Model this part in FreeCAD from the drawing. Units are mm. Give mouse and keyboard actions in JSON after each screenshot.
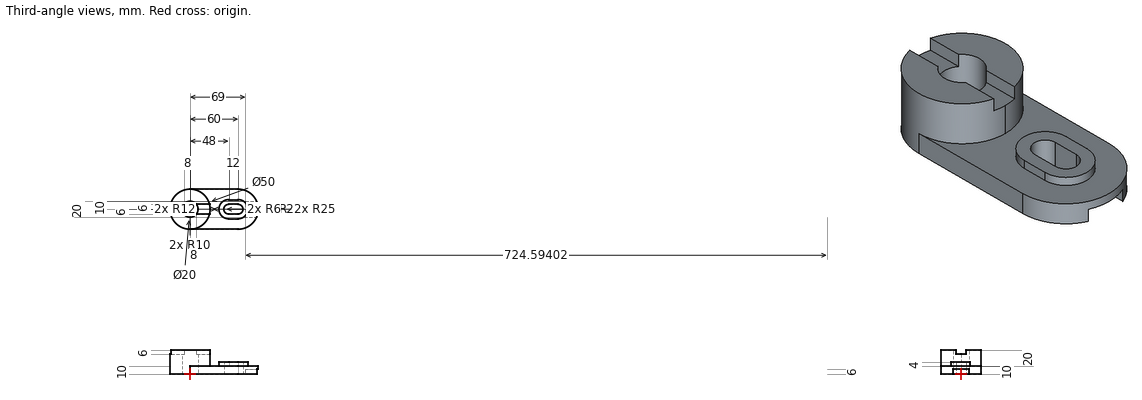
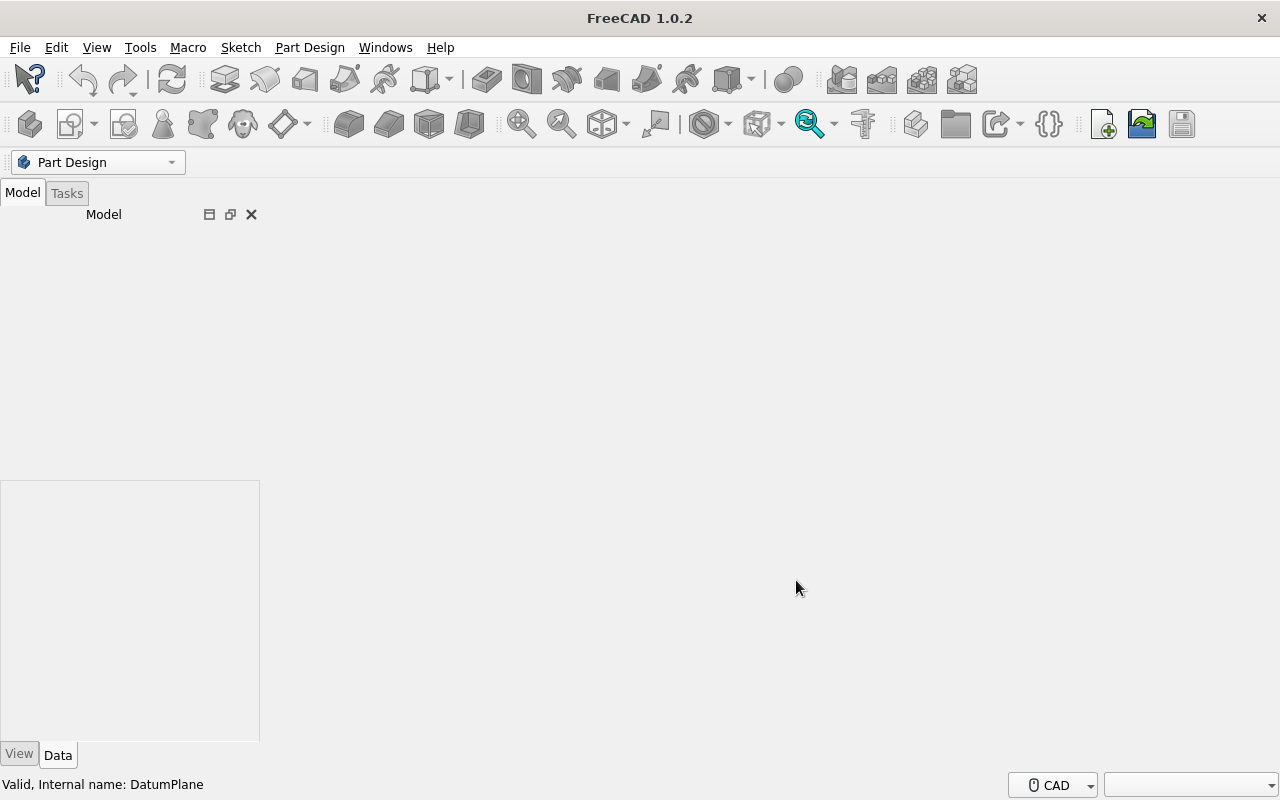
{"action": "left_click", "coordinate": [1102, 124]}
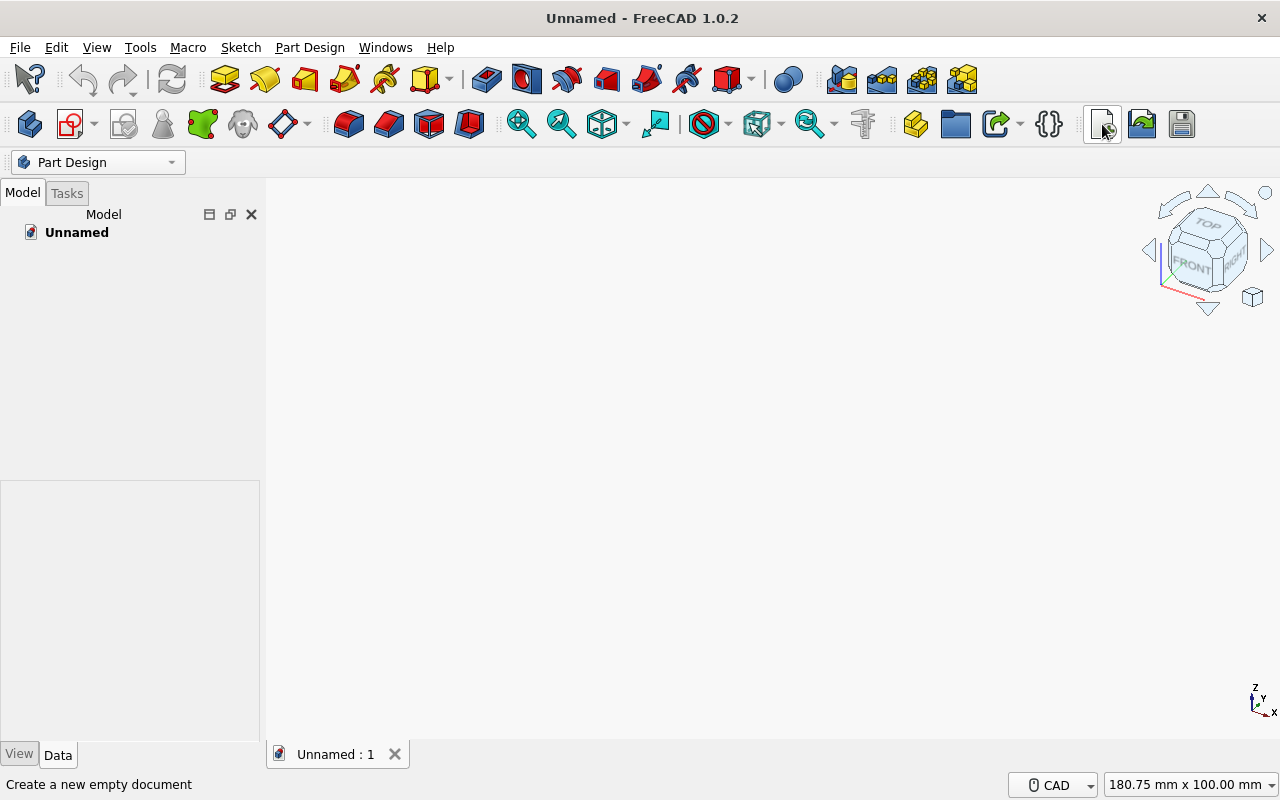
{"action": "left_click", "coordinate": [70, 124]}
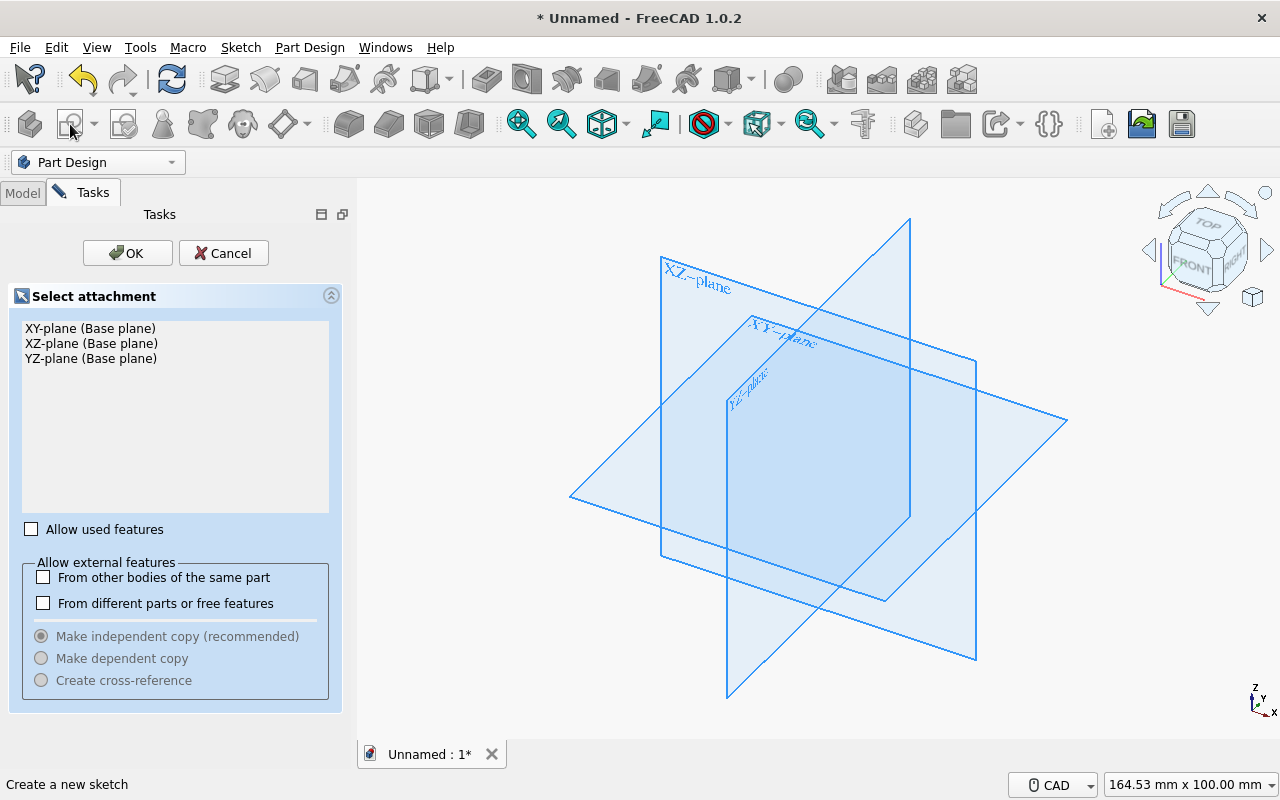
{"action": "left_click", "coordinate": [82, 328]}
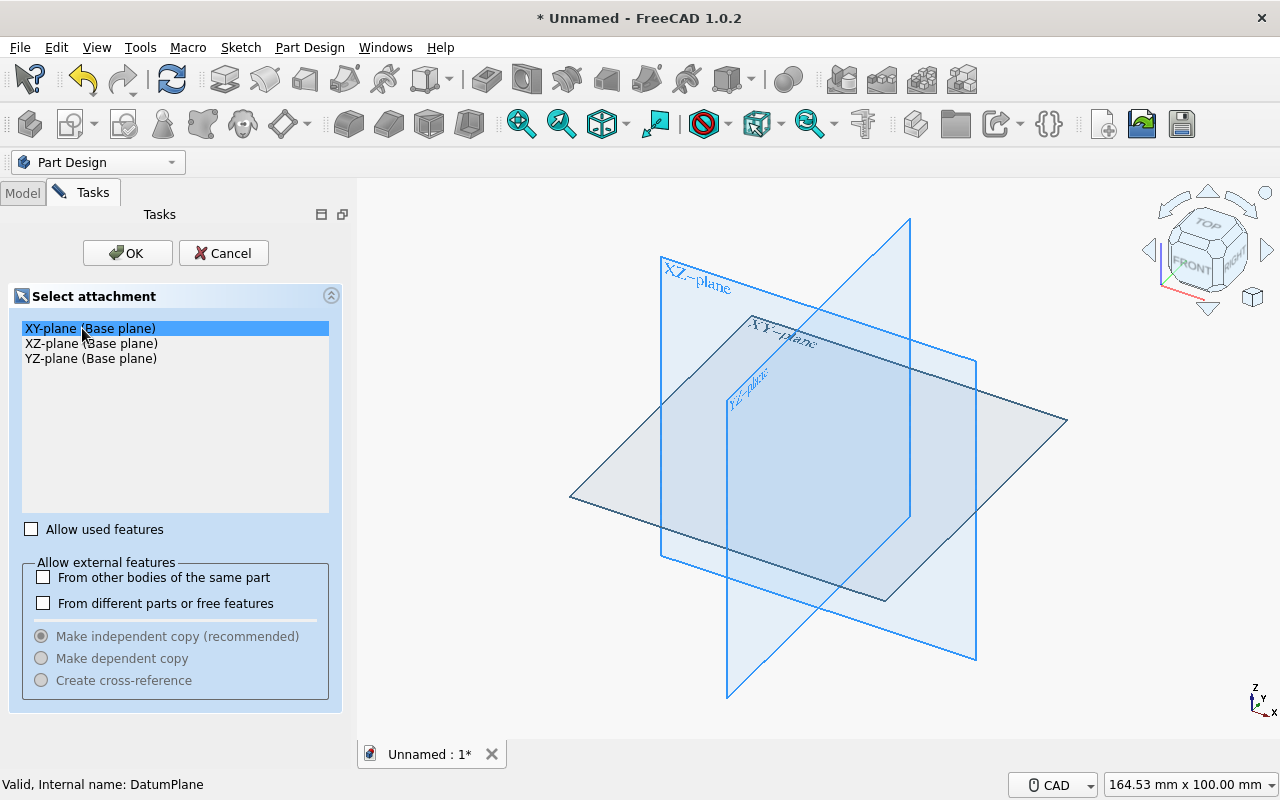
{"action": "left_click", "coordinate": [128, 253]}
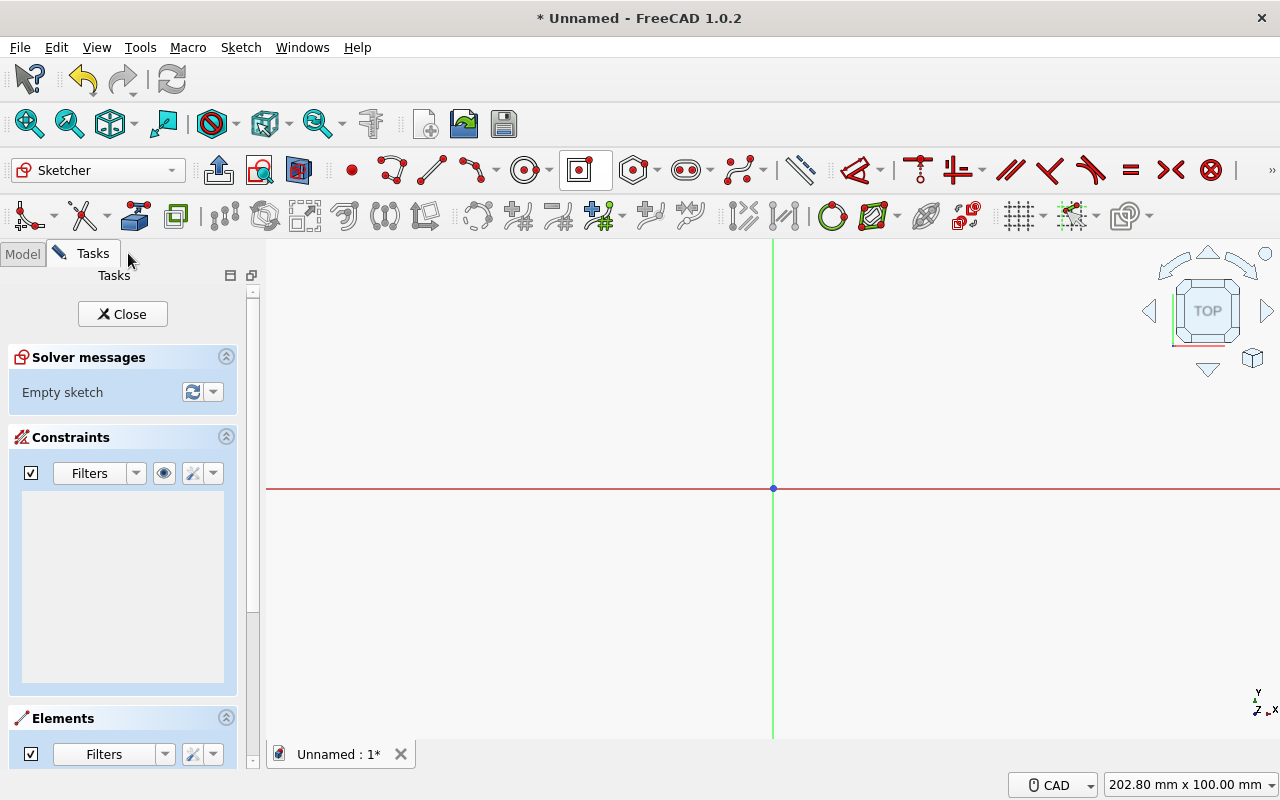
{"action": "scroll", "coordinate": [294, 489], "scroll_direction": "down", "scroll_amount": 1}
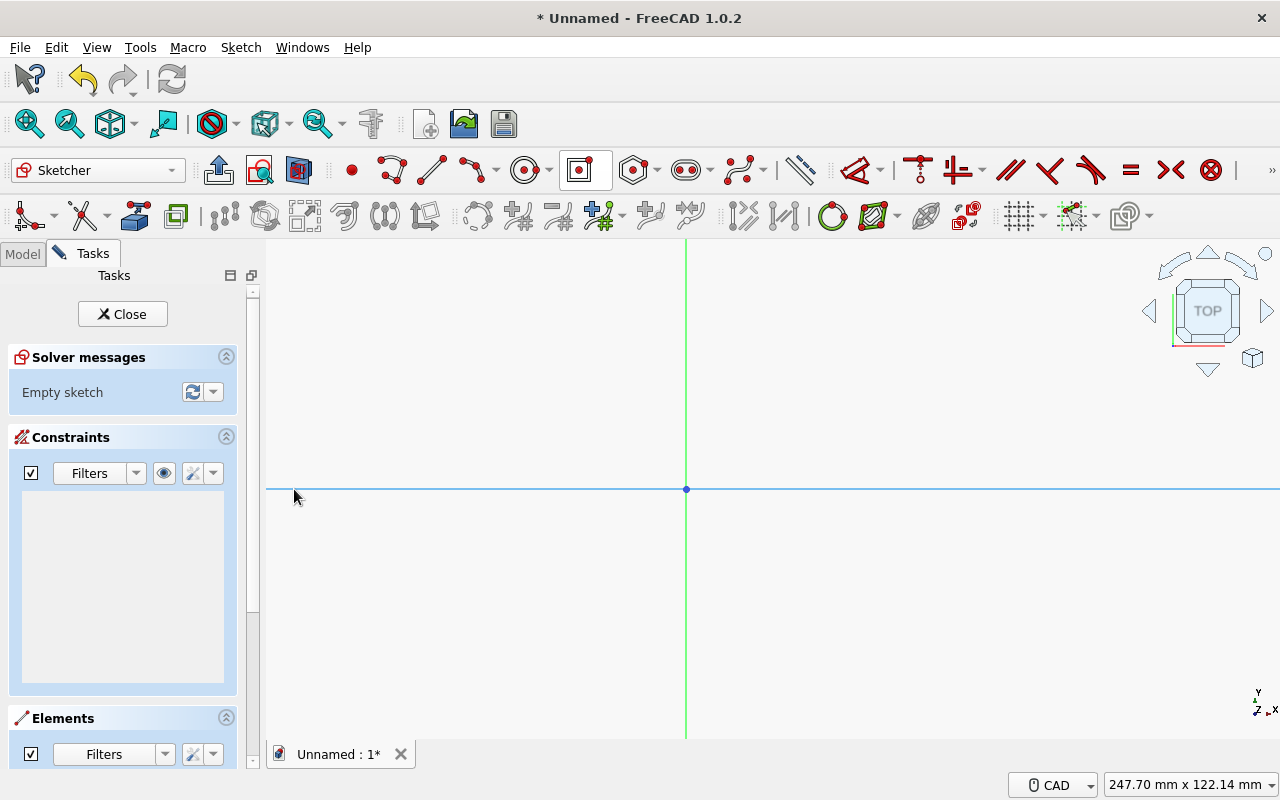
{"action": "scroll", "coordinate": [1115, 489], "scroll_direction": "up", "scroll_amount": 2}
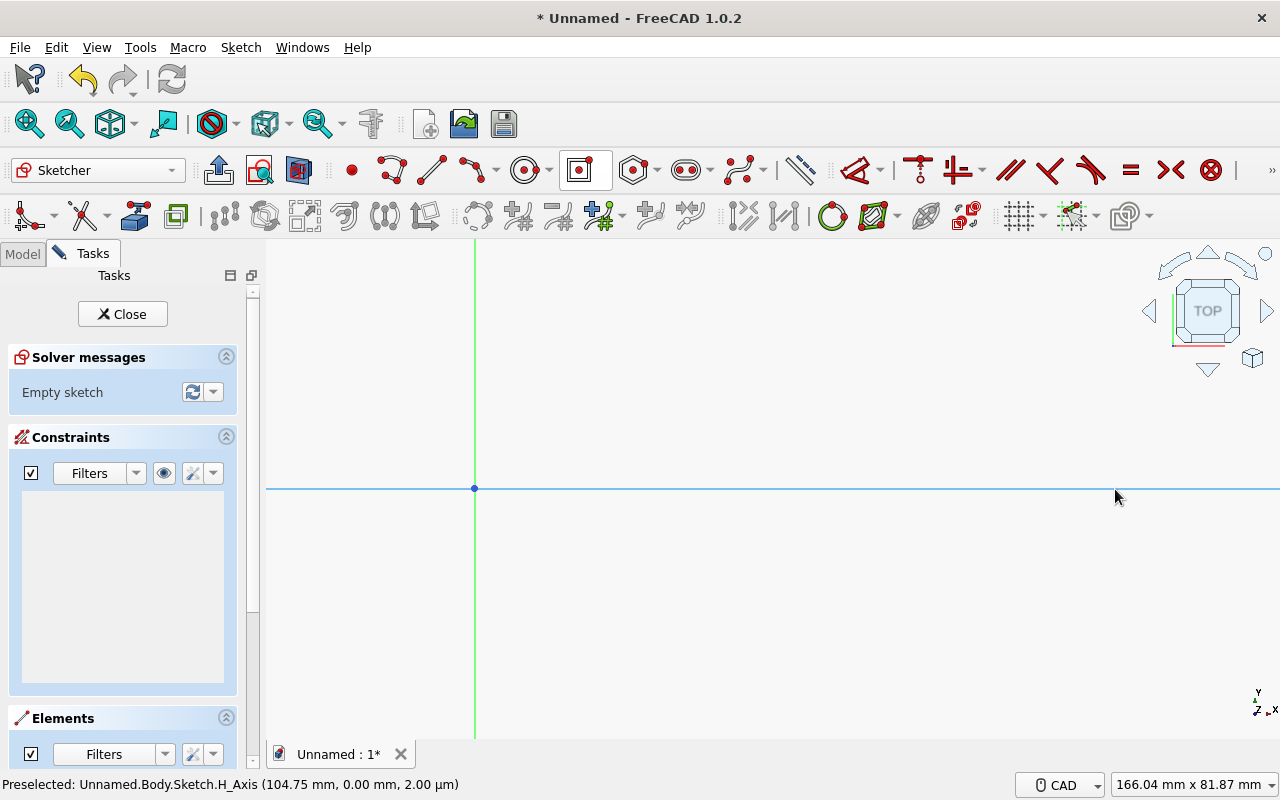
{"action": "left_click", "coordinate": [392, 170]}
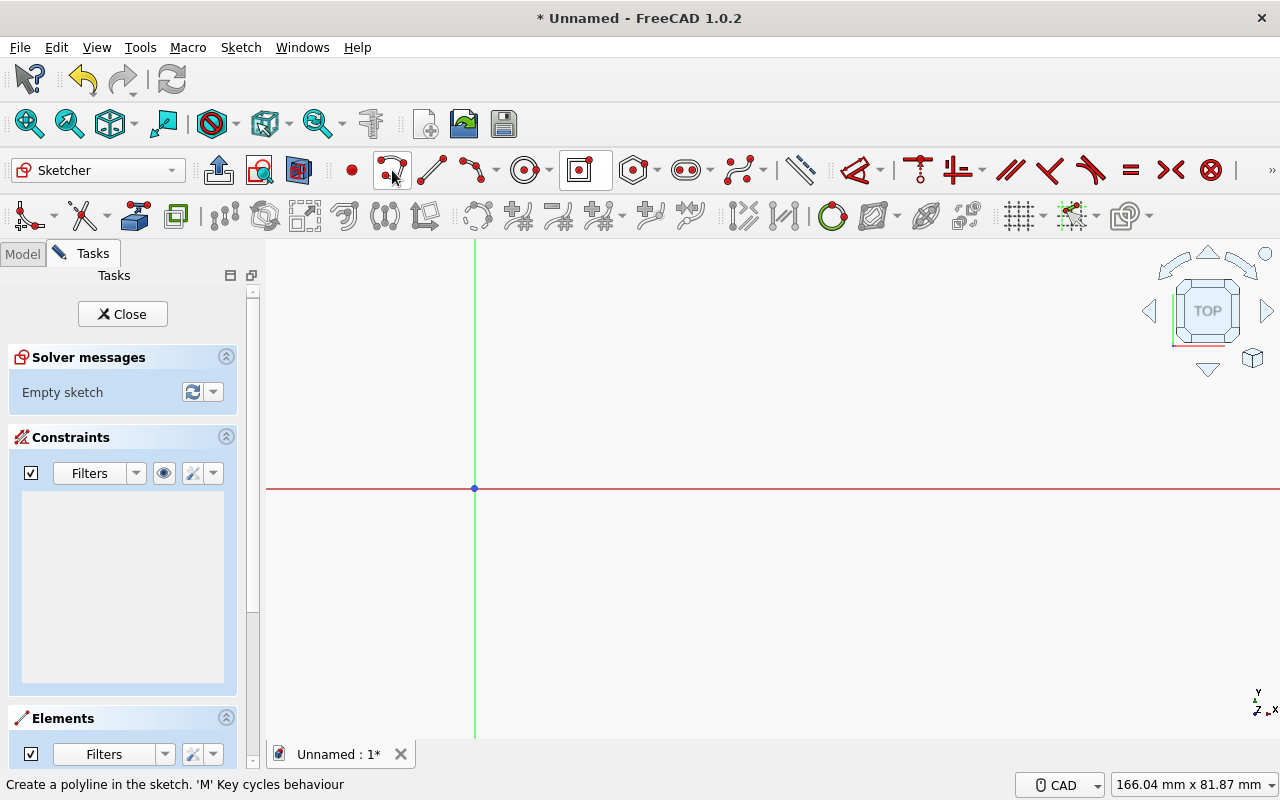
{"action": "left_click", "coordinate": [841, 336]}
{"action": "left_click", "coordinate": [475, 336]}
{"action": "left_click", "coordinate": [484, 642]}
{"action": "left_click", "coordinate": [841, 642]}
{"action": "right_click", "coordinate": [841, 642]}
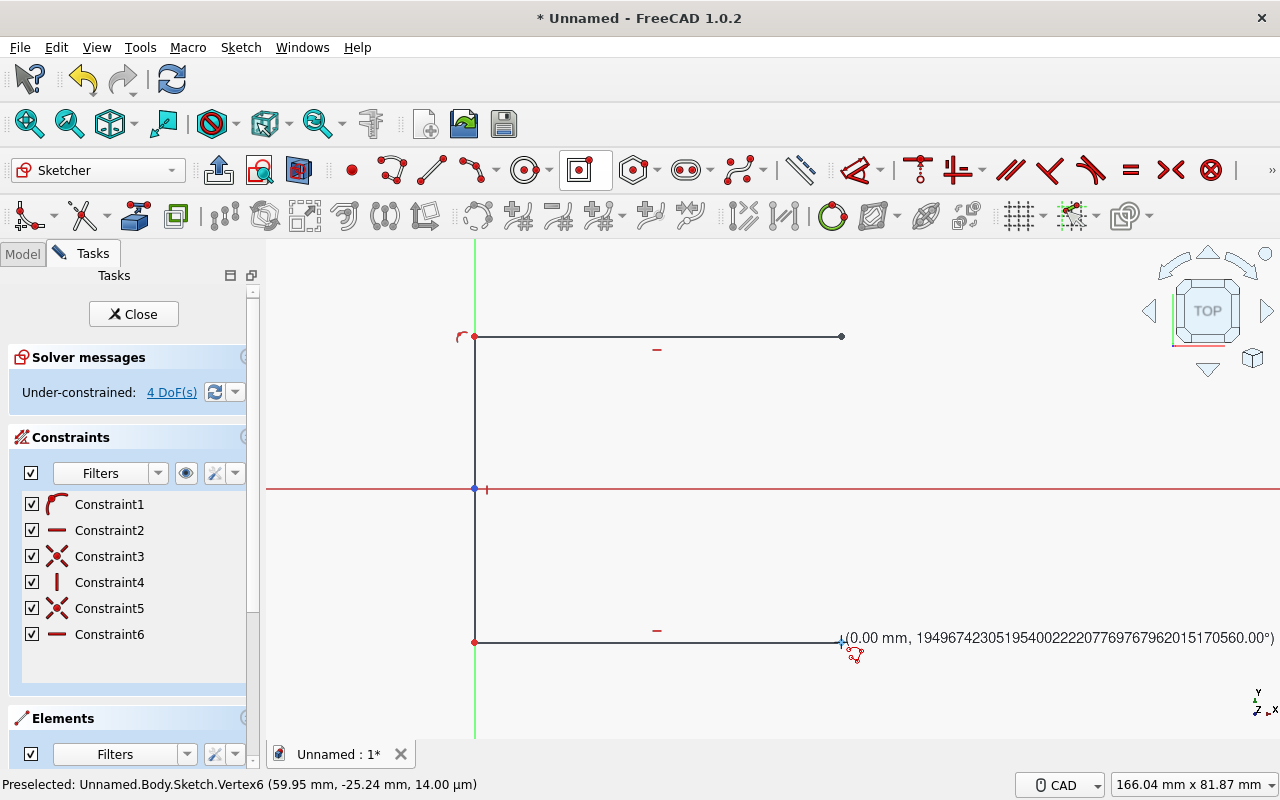
{"action": "left_click", "coordinate": [472, 170]}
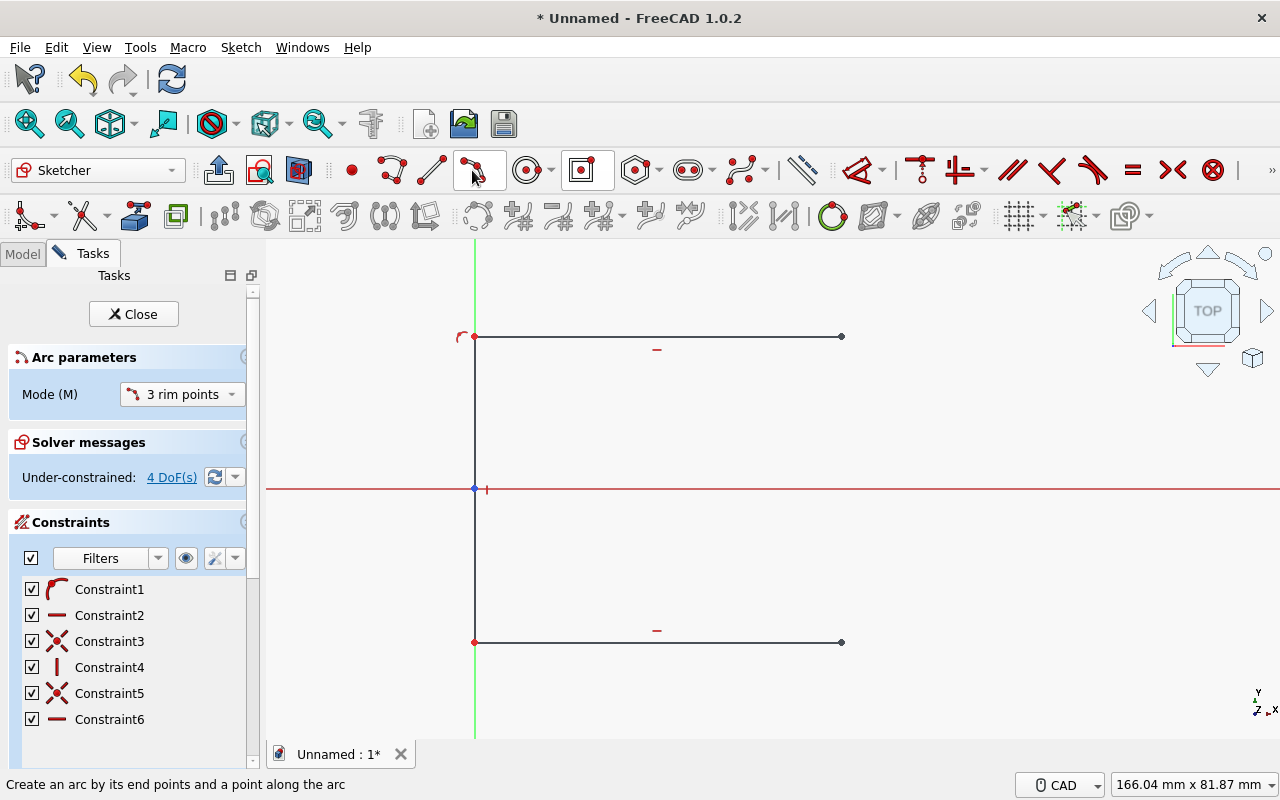
{"action": "left_click", "coordinate": [841, 643]}
{"action": "left_click", "coordinate": [841, 337]}
{"action": "left_click", "coordinate": [986, 536]}
{"action": "key", "text": "Escape"}